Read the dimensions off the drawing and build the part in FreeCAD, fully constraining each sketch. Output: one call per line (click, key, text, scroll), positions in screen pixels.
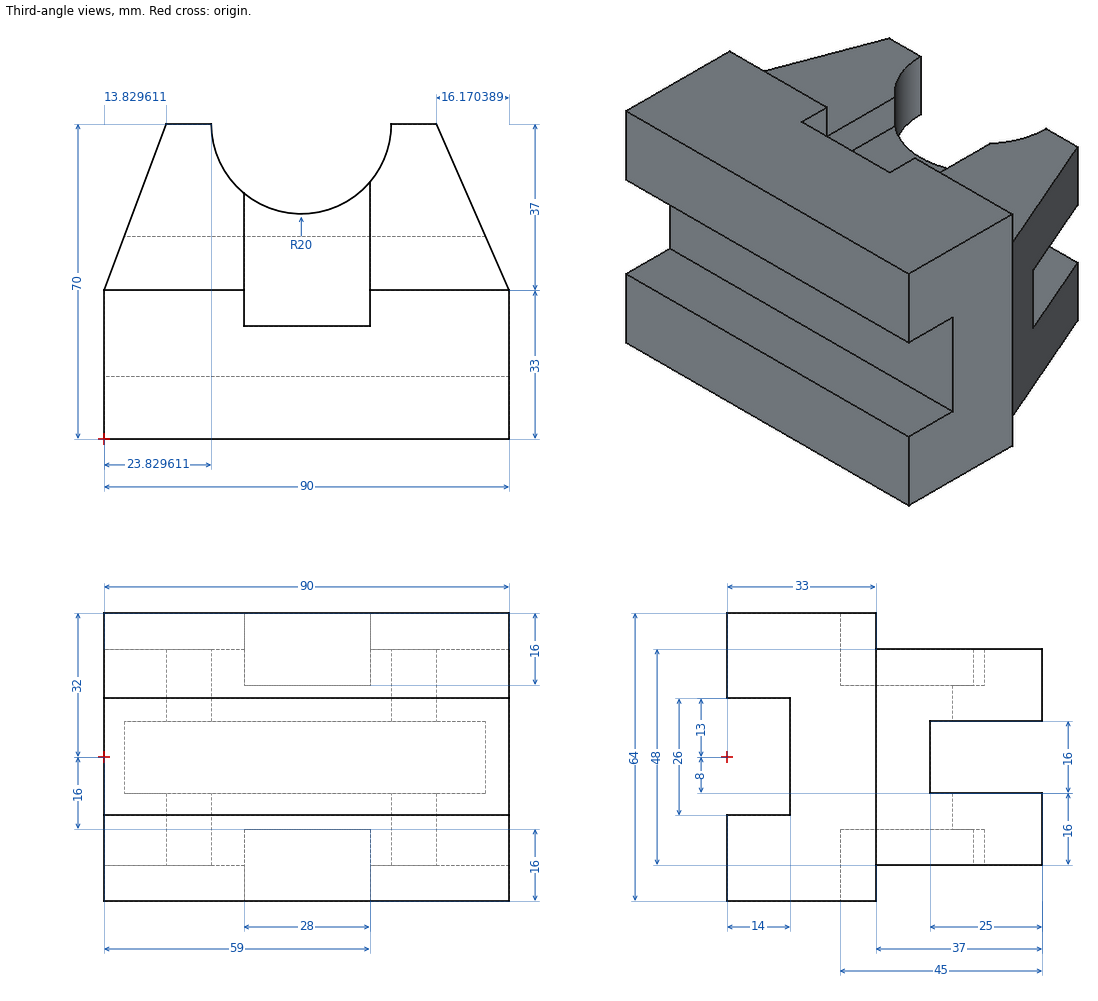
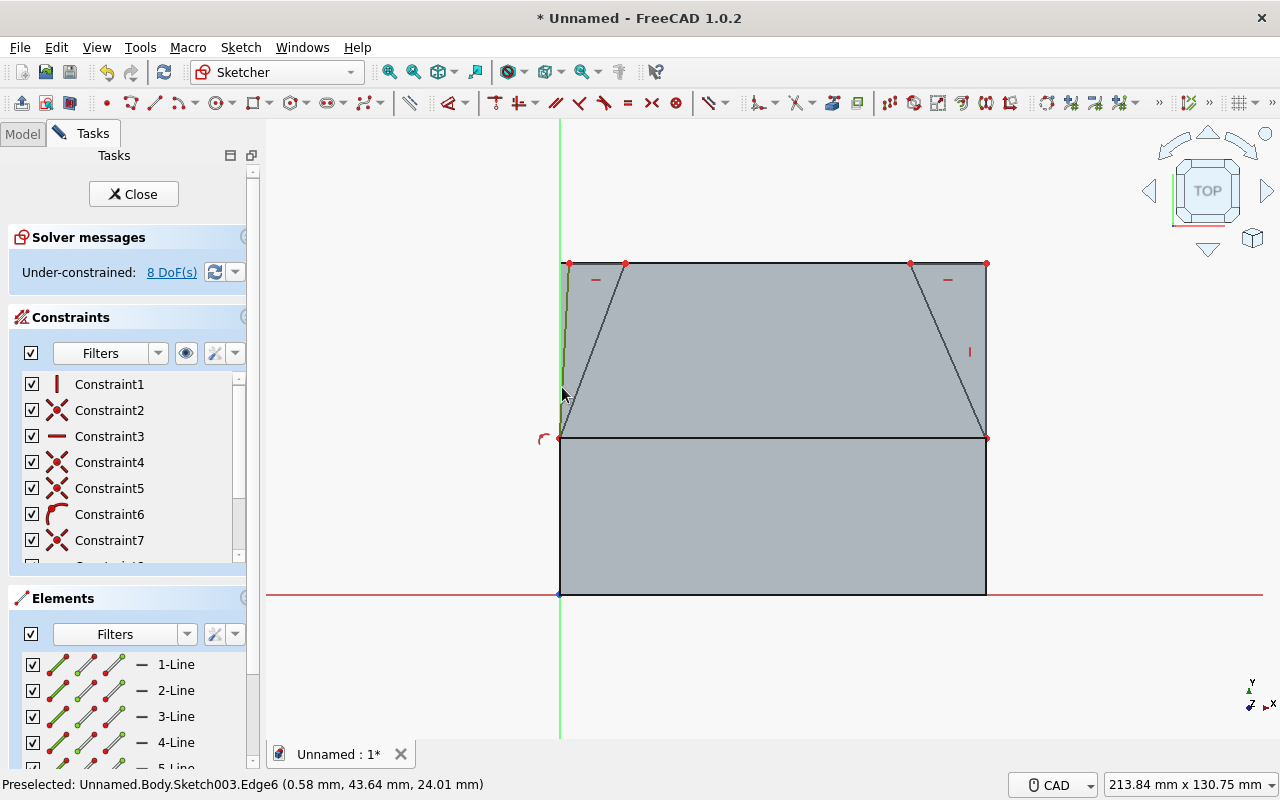
click(538, 104)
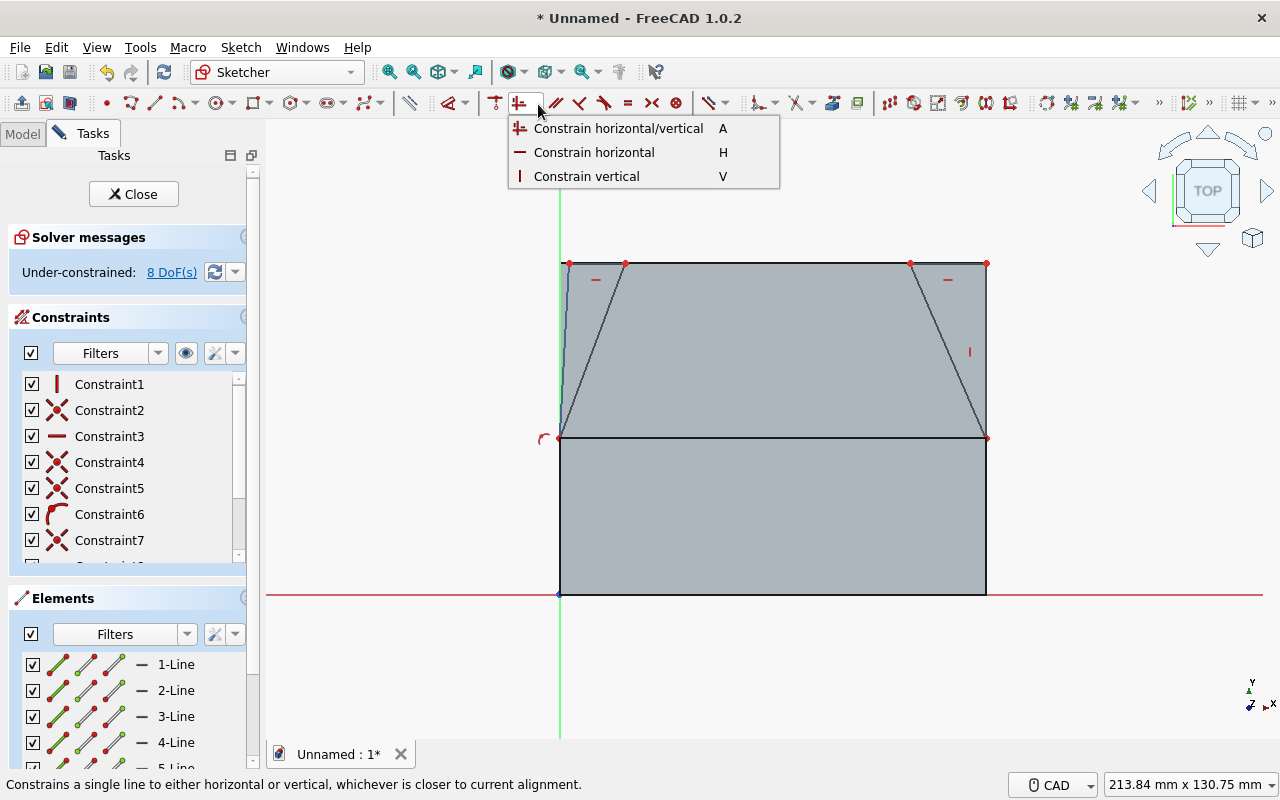
click(644, 176)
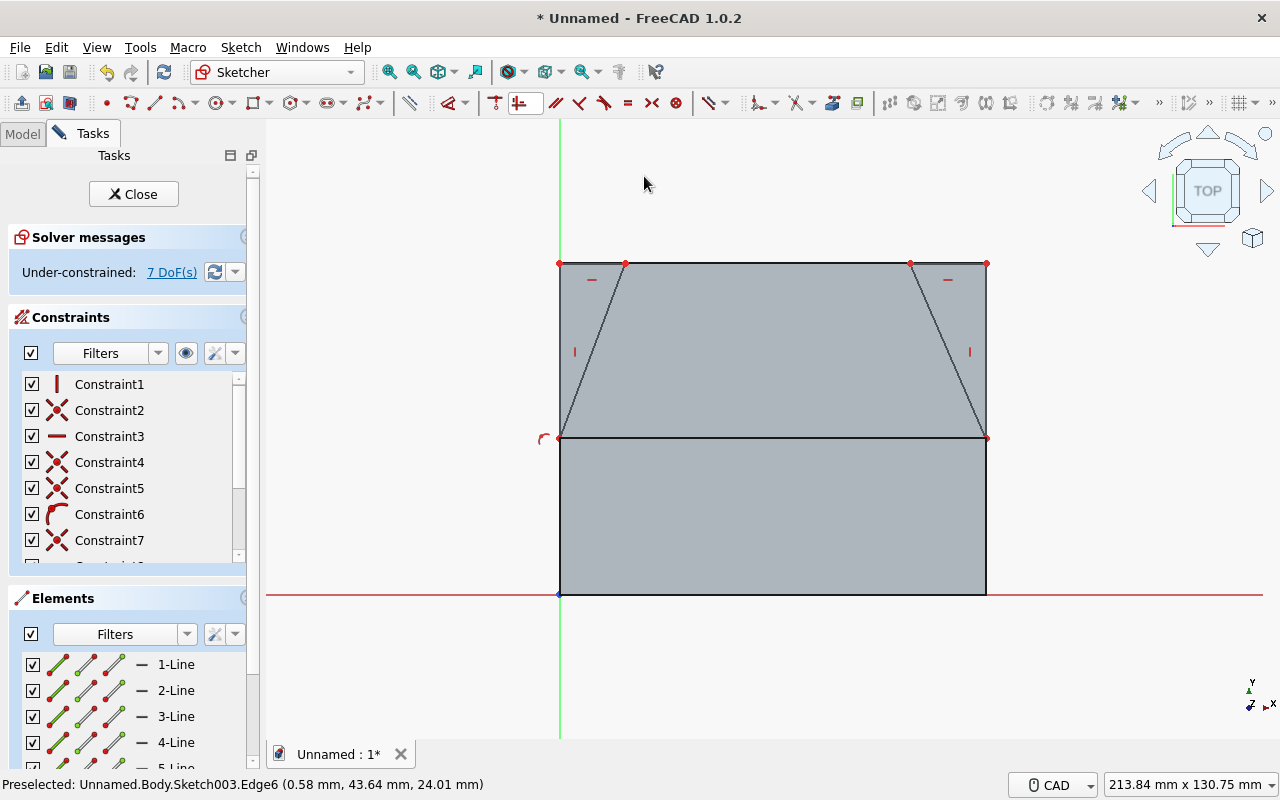
click(448, 104)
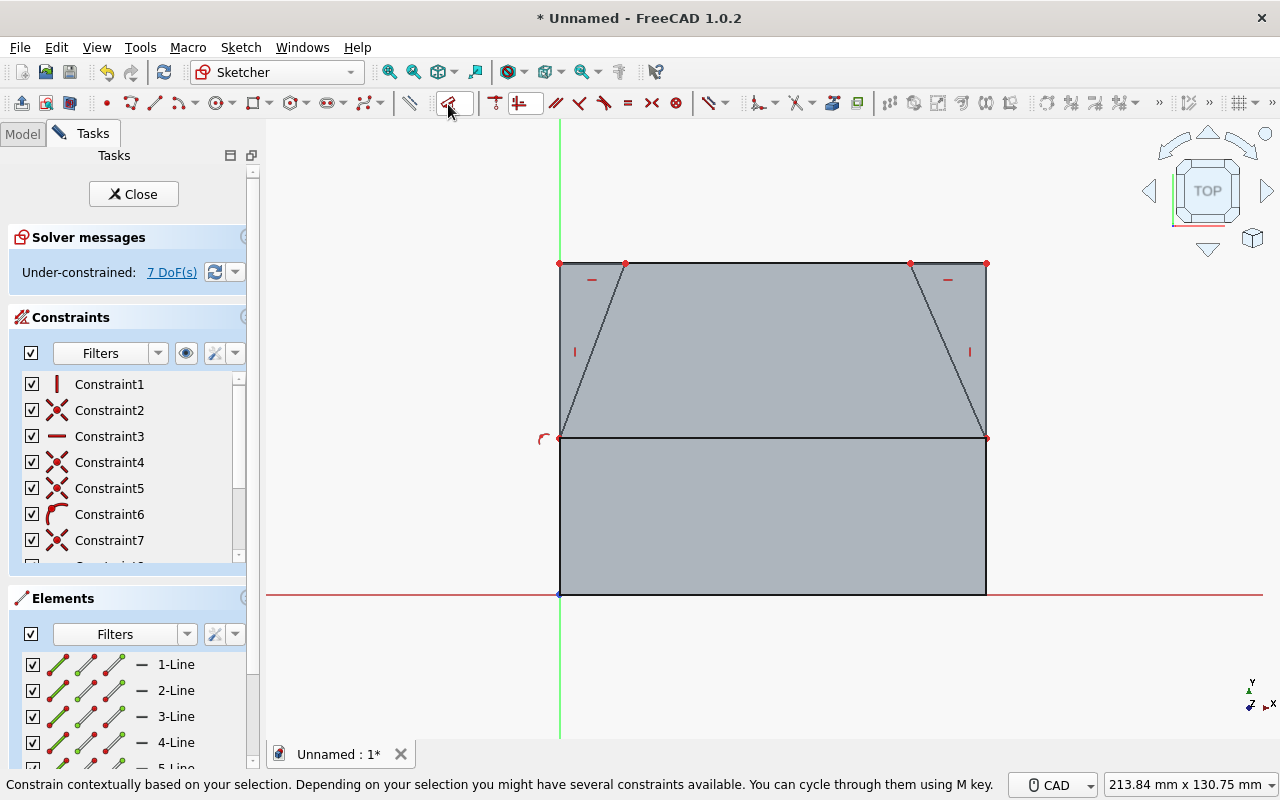
click(986, 387)
click(1020, 352)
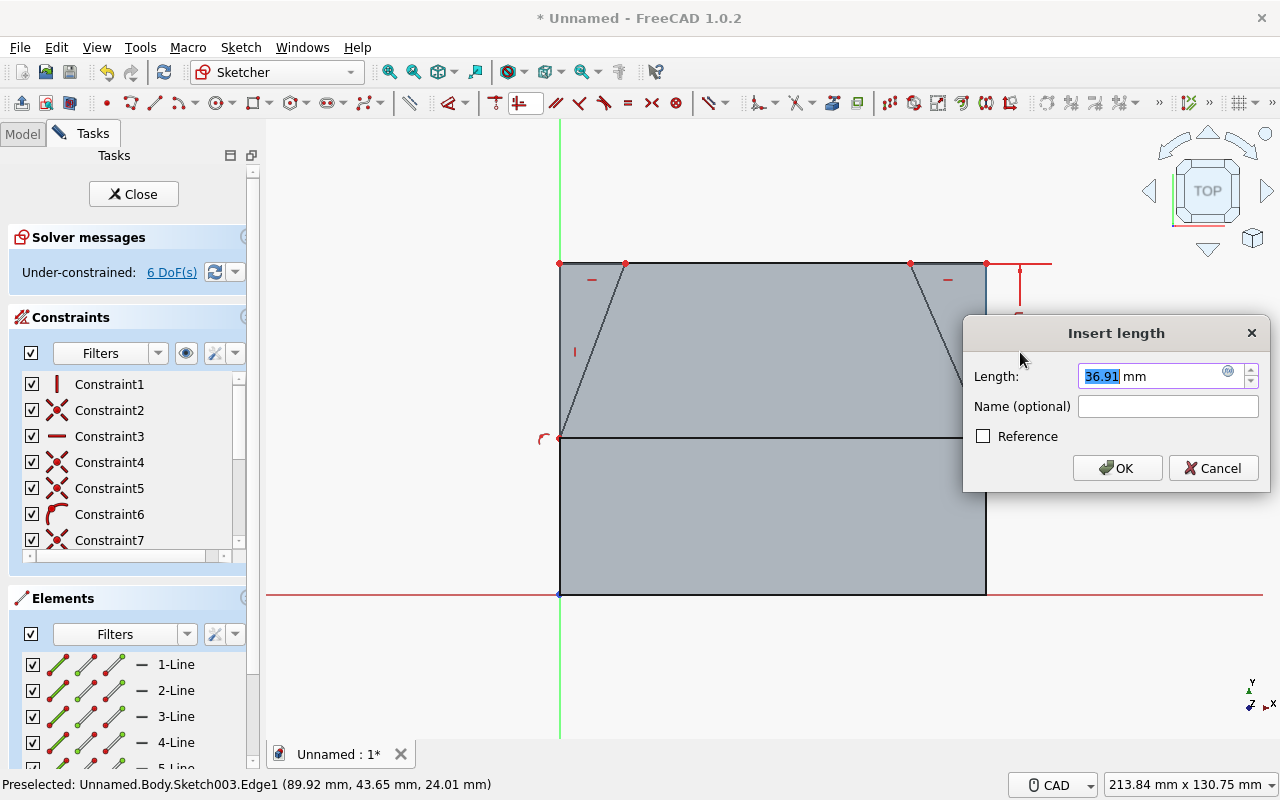
text(37)
key(Return)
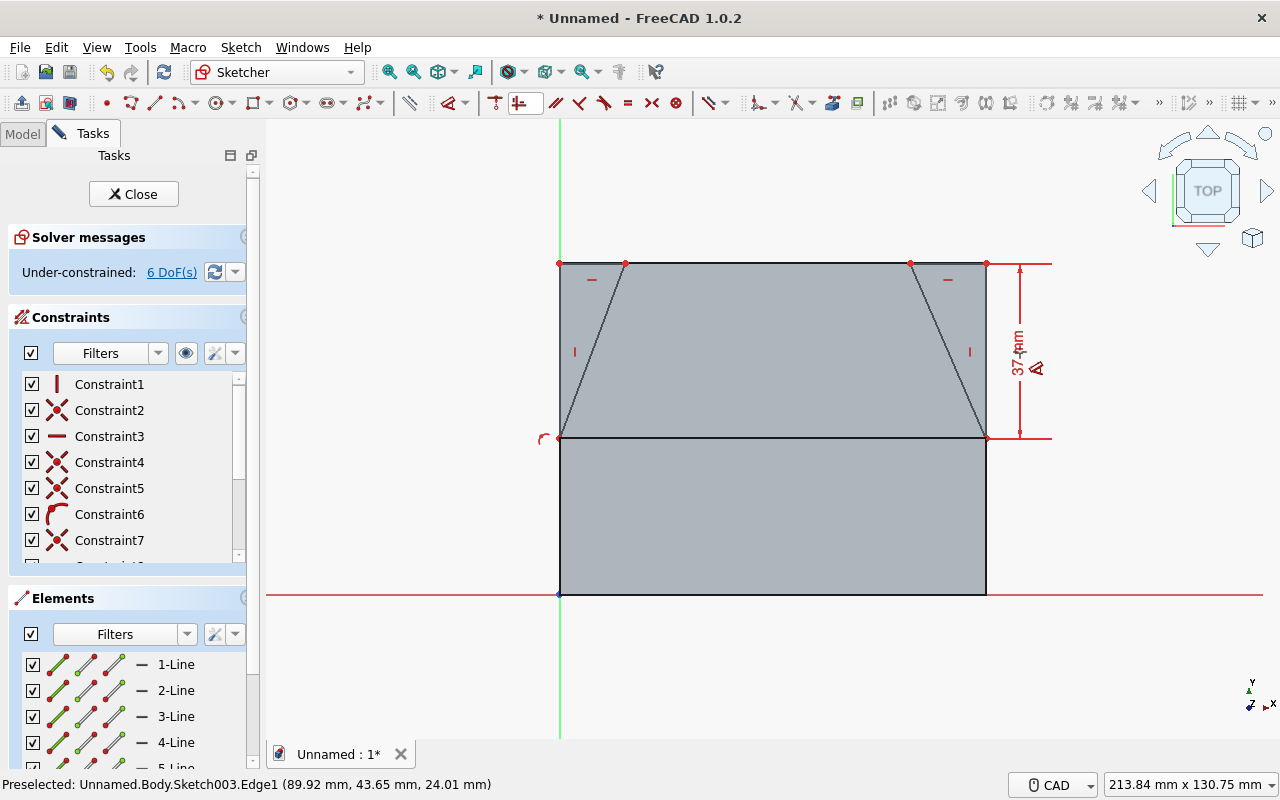
click(560, 317)
click(526, 352)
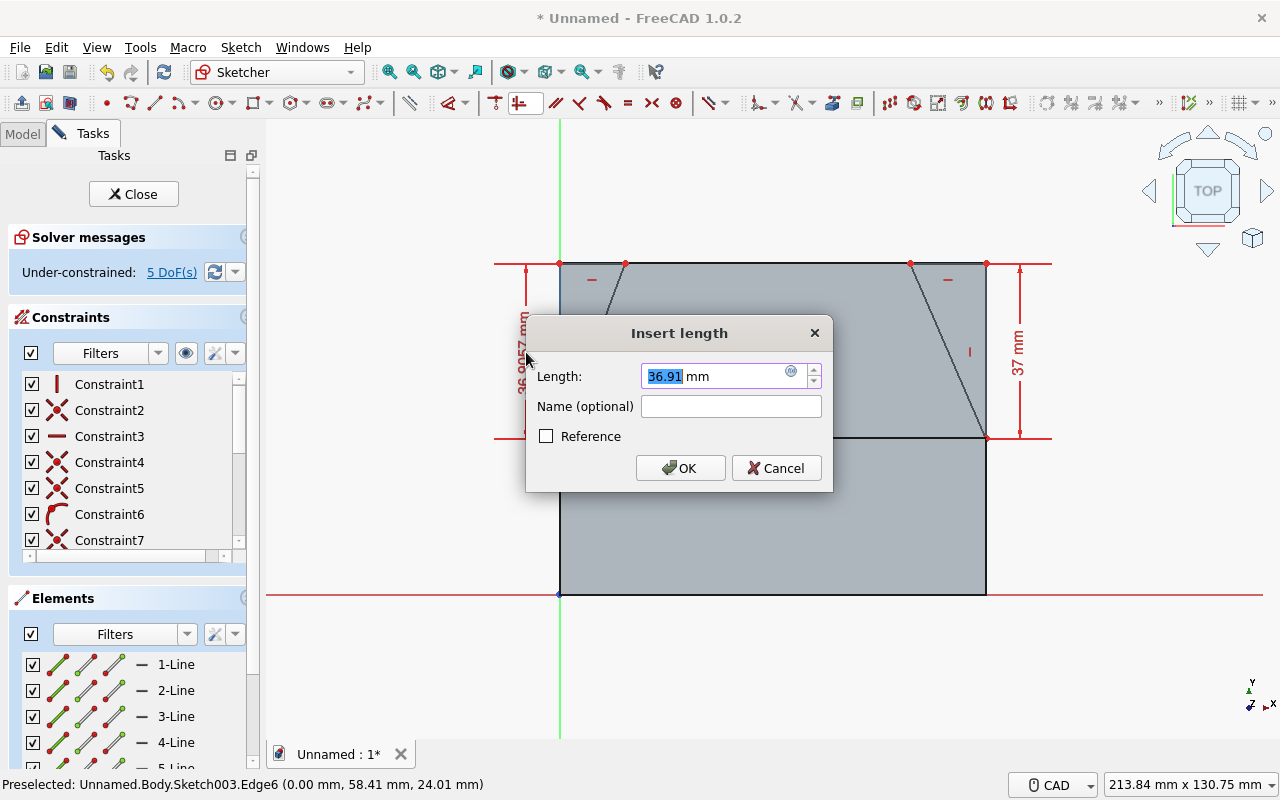
text(37)
key(Return)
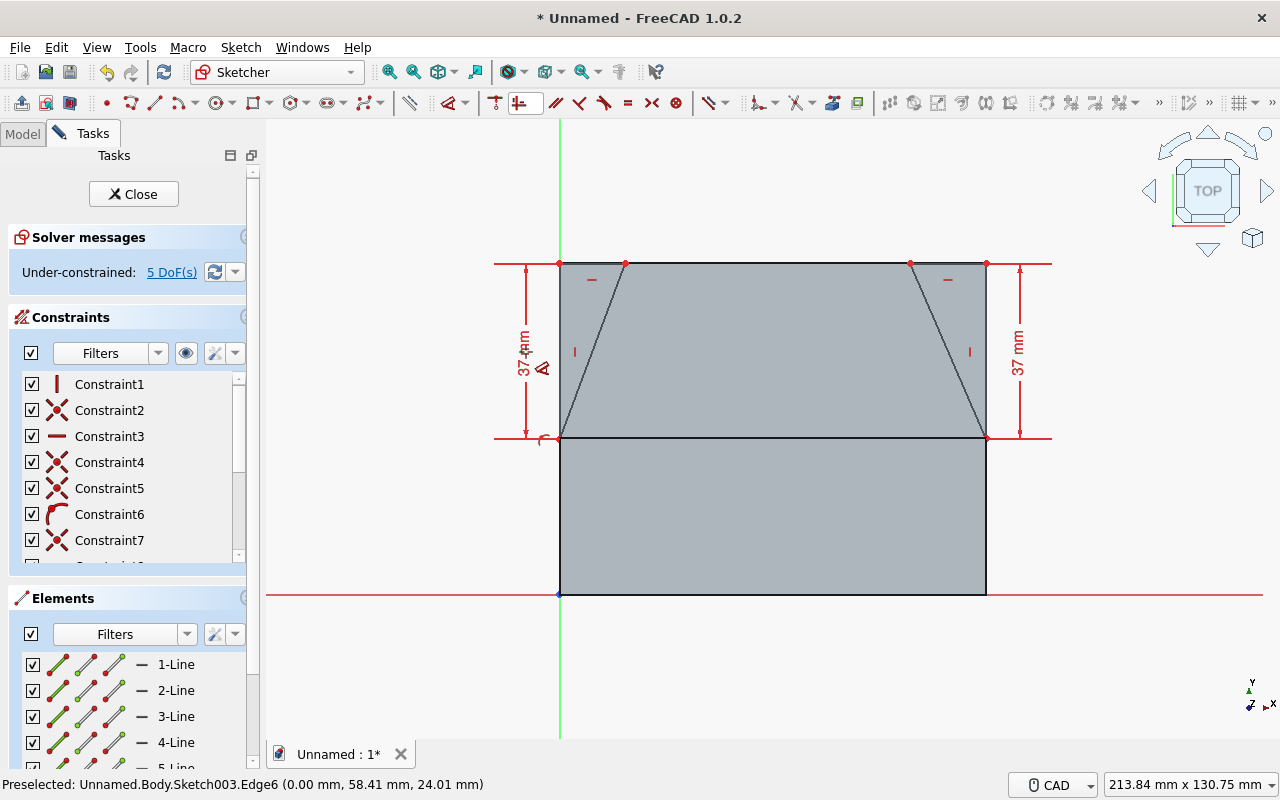
click(986, 439)
click(773, 629)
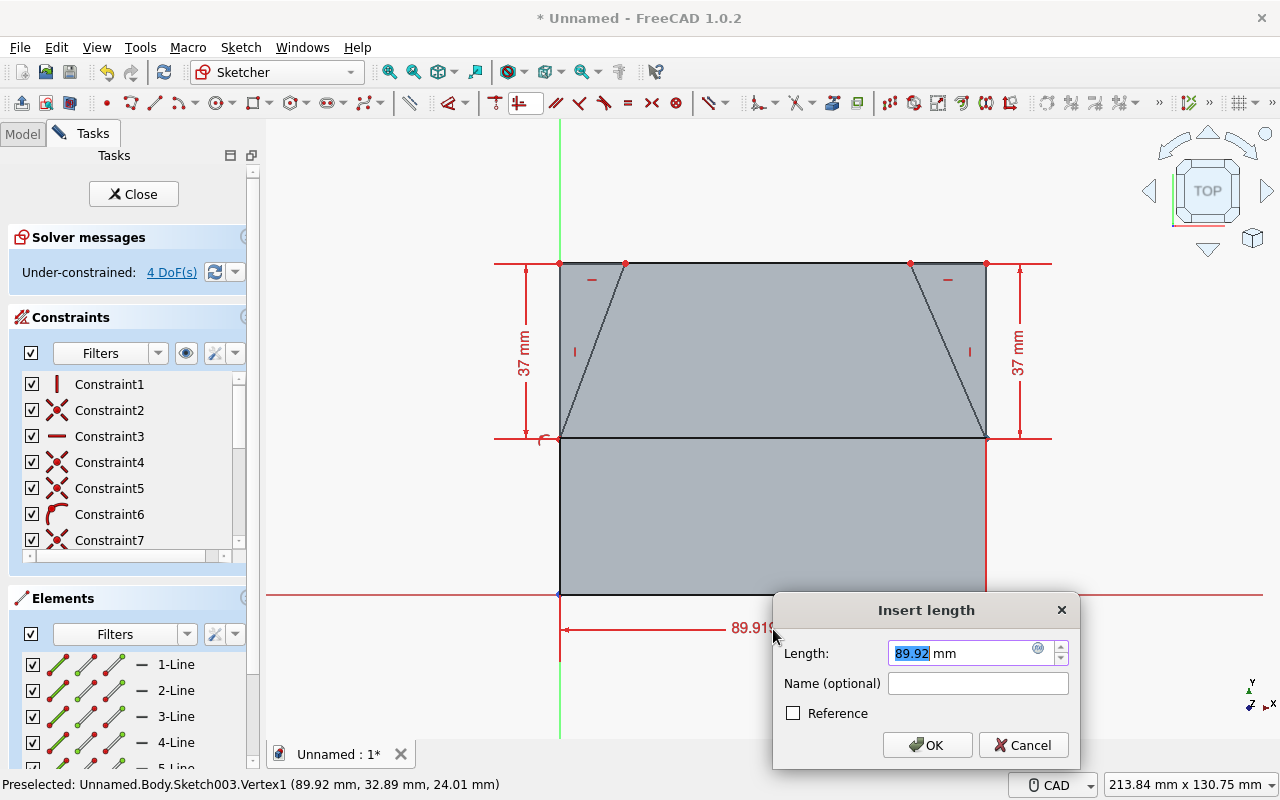
text(90)
key(Return)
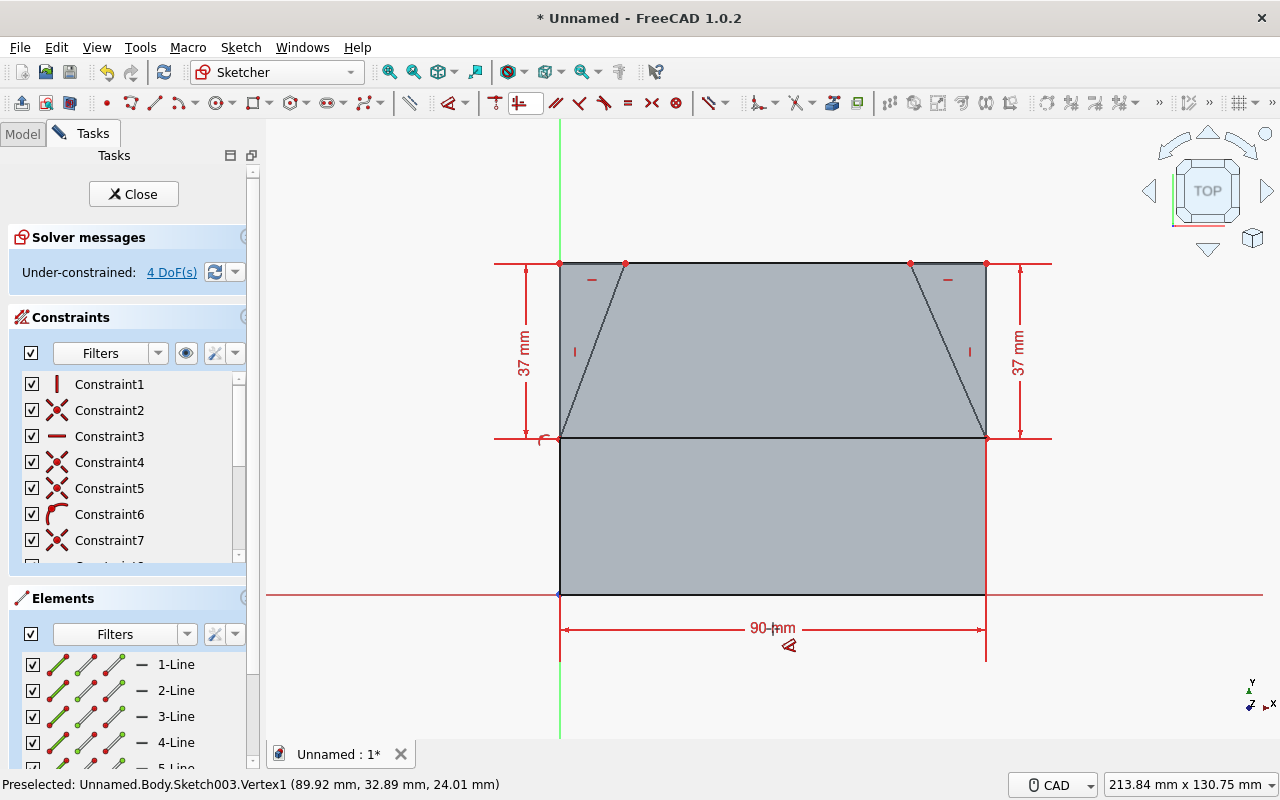
click(986, 439)
click(1020, 517)